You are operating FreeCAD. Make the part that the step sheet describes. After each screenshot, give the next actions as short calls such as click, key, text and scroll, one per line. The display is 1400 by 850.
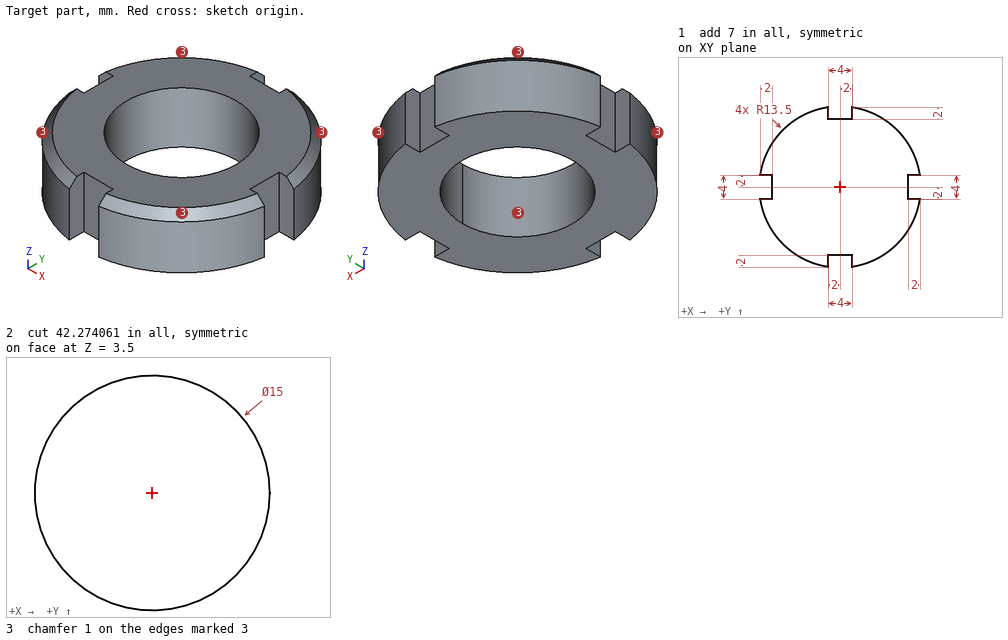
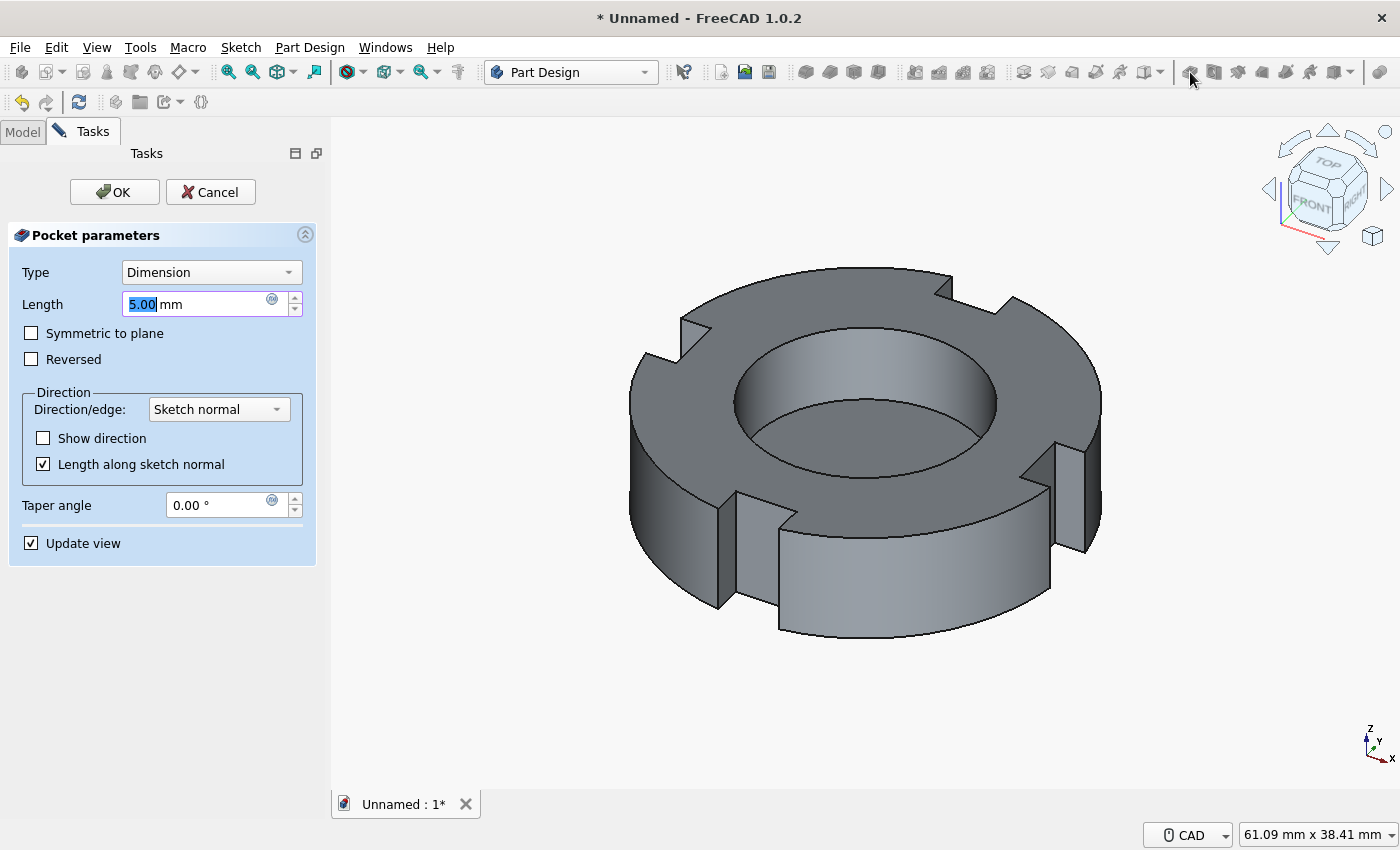
text(42.274061)
key(Tab)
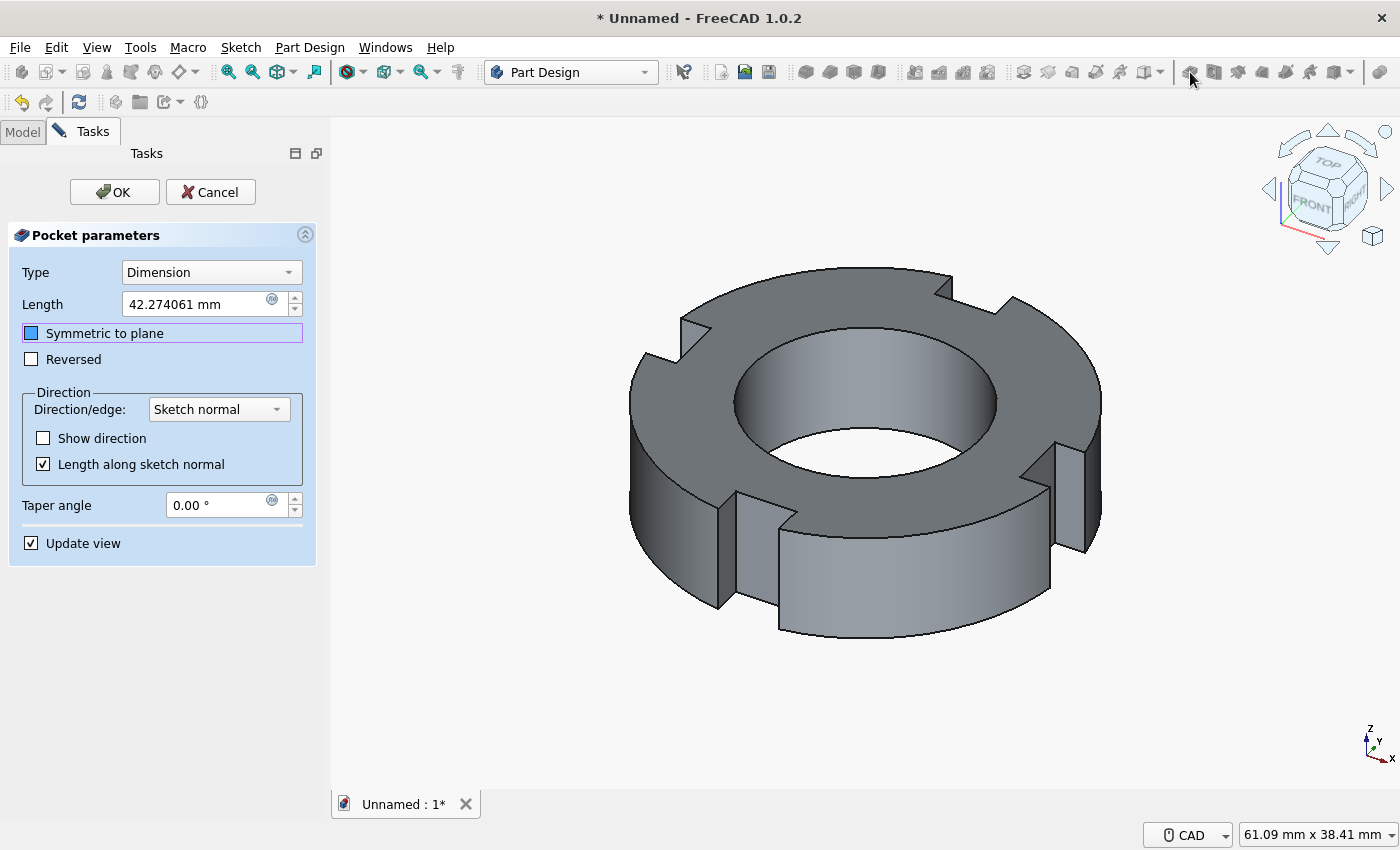
click(30, 333)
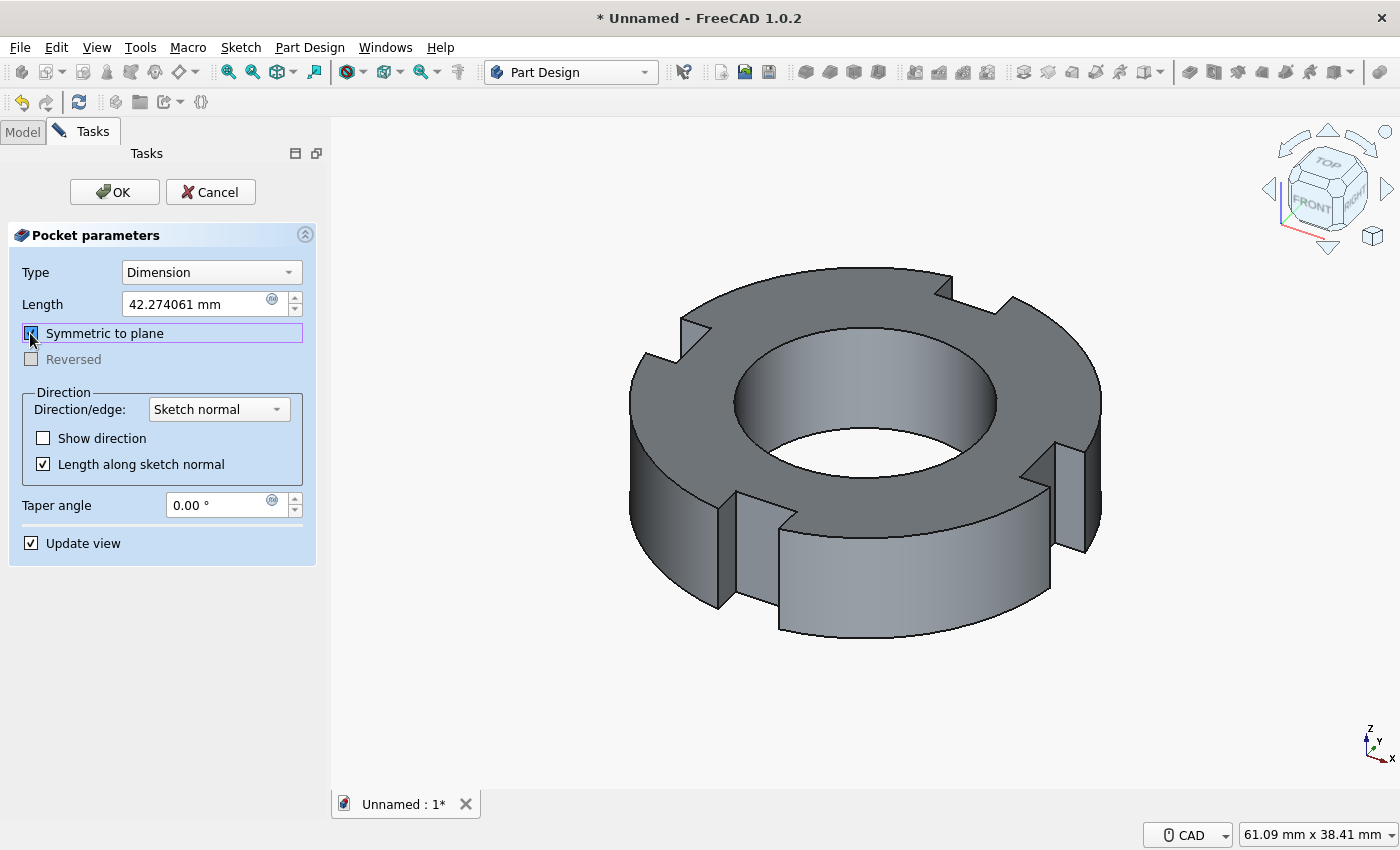
click(115, 192)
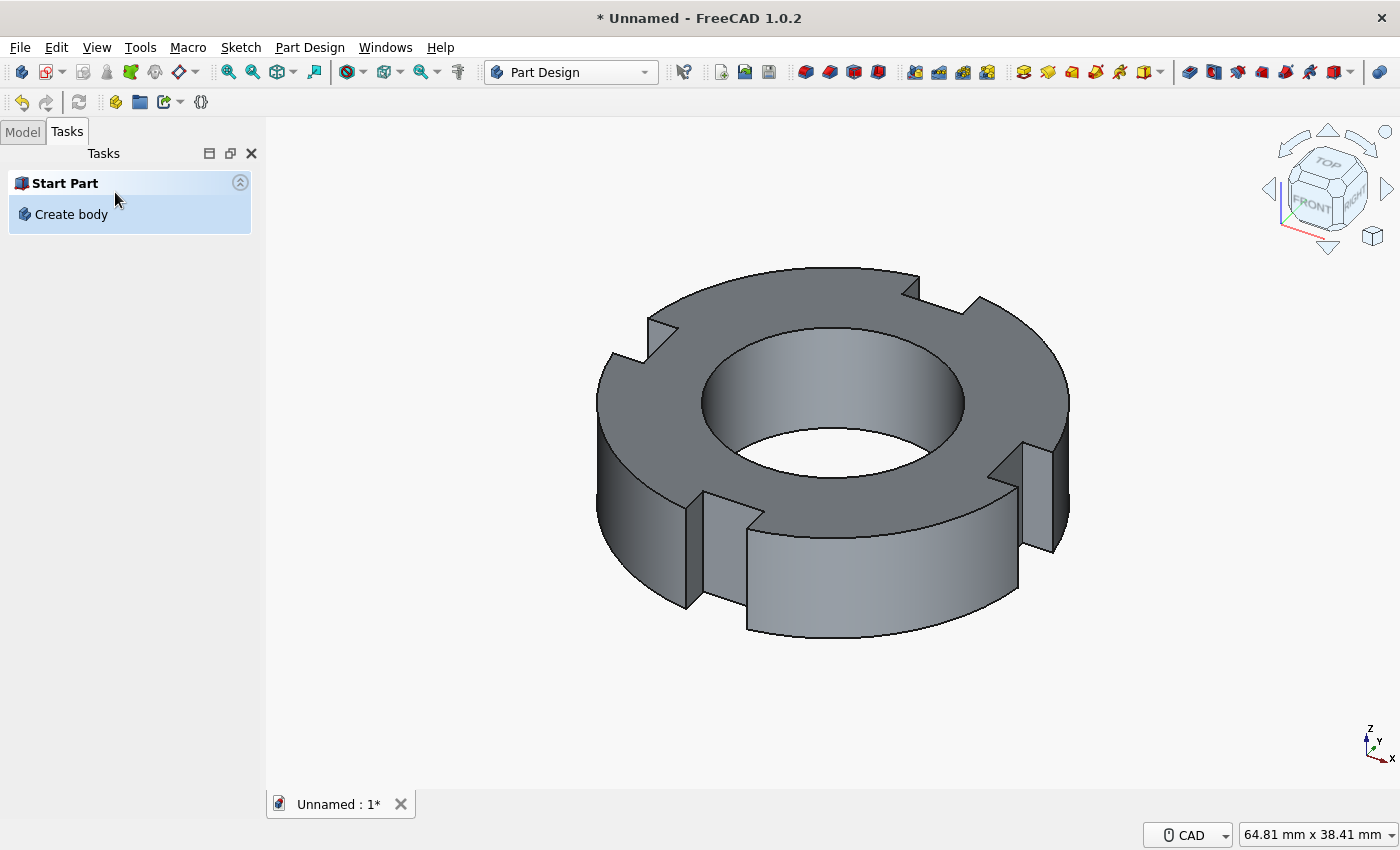
click(605, 437)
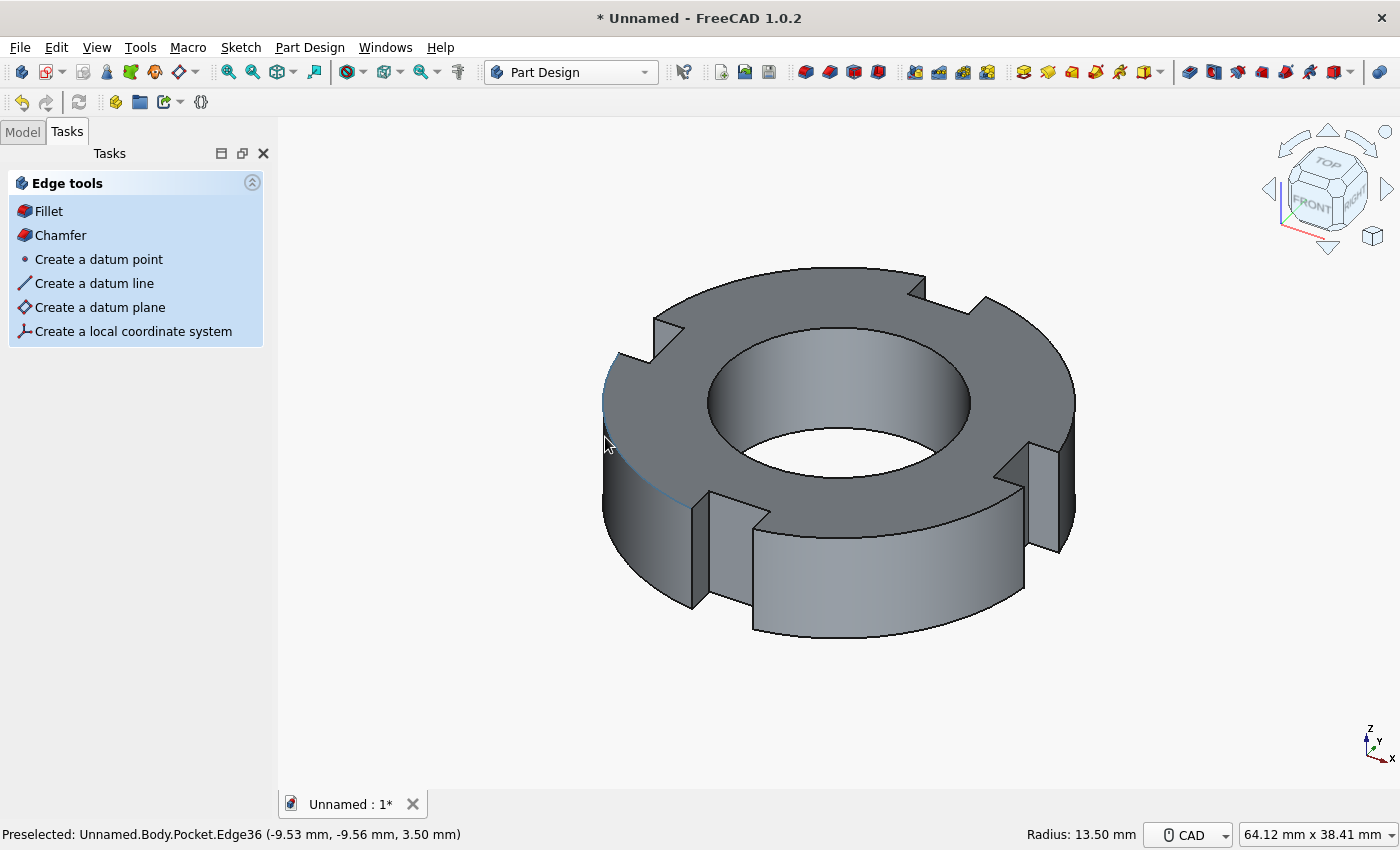
click(900, 533, ctrl)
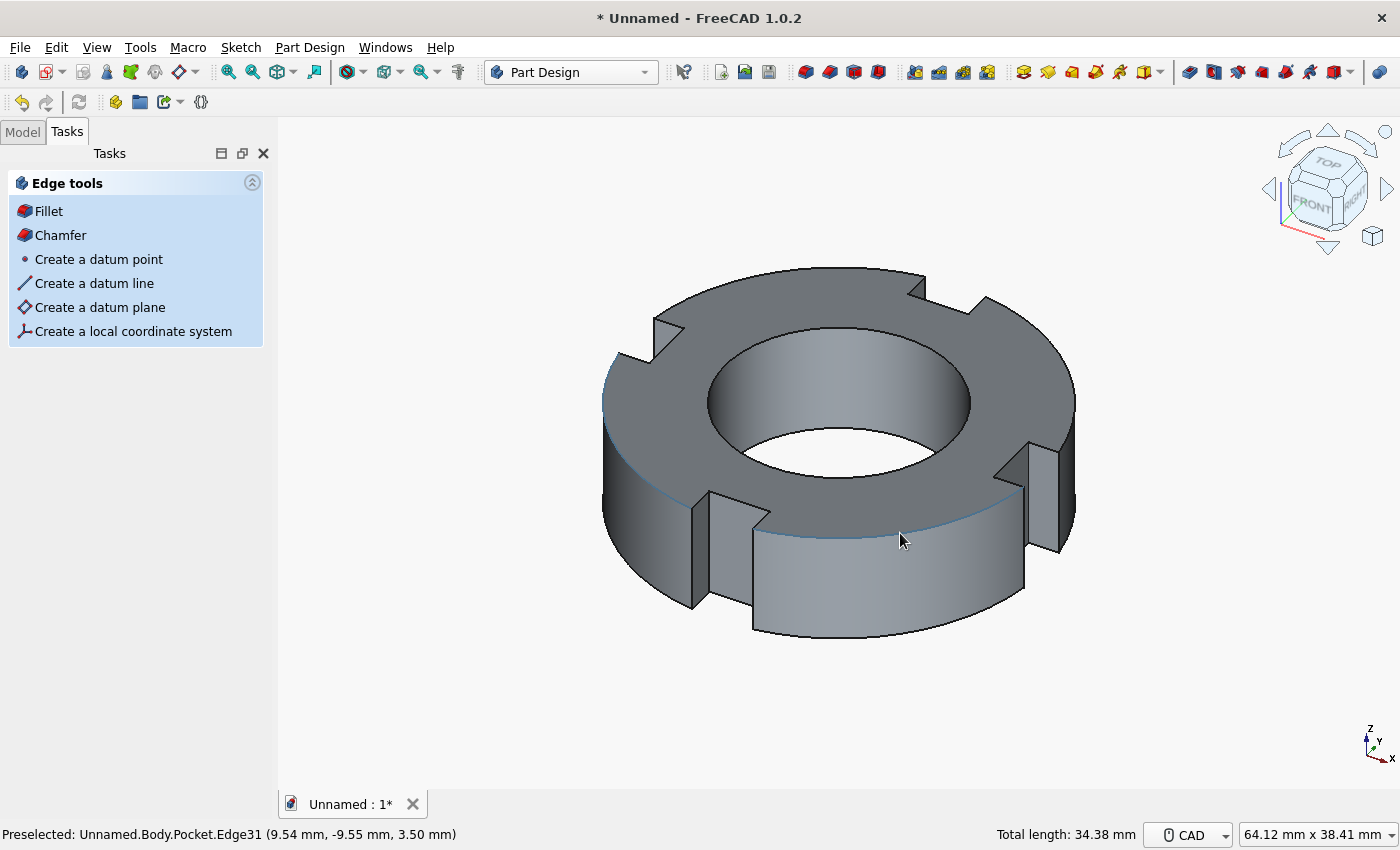
click(1058, 350, ctrl)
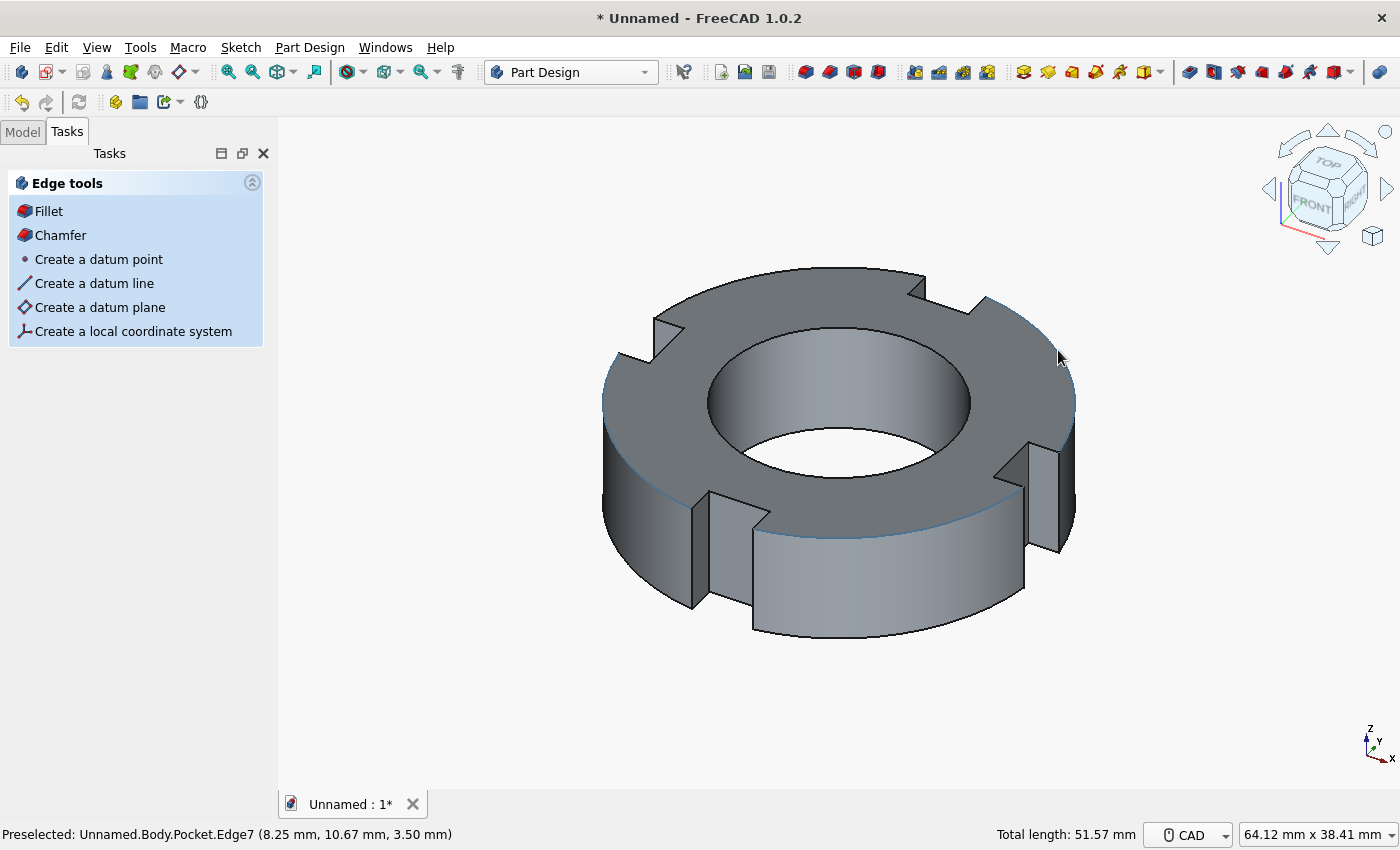
key(0)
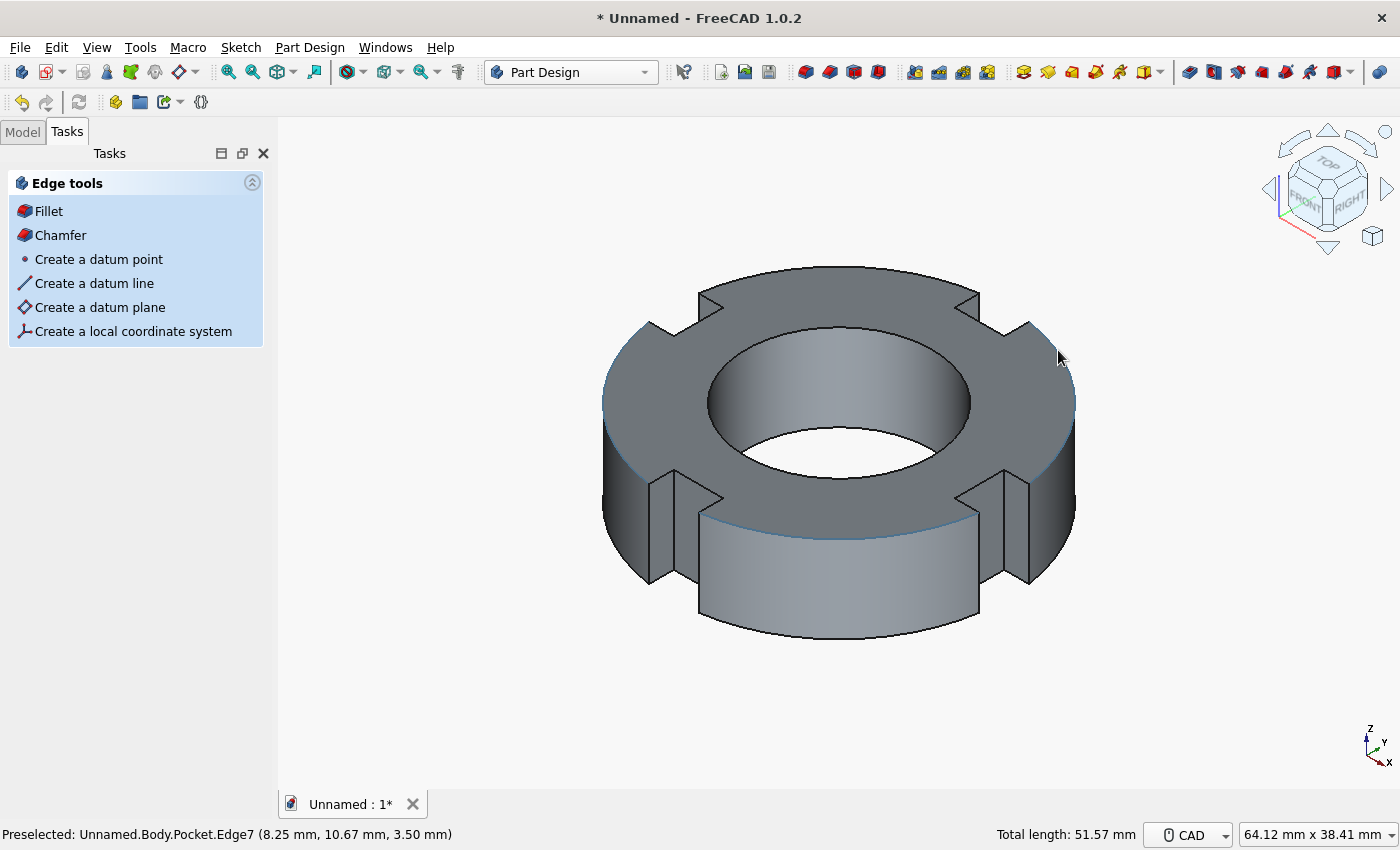
key(2)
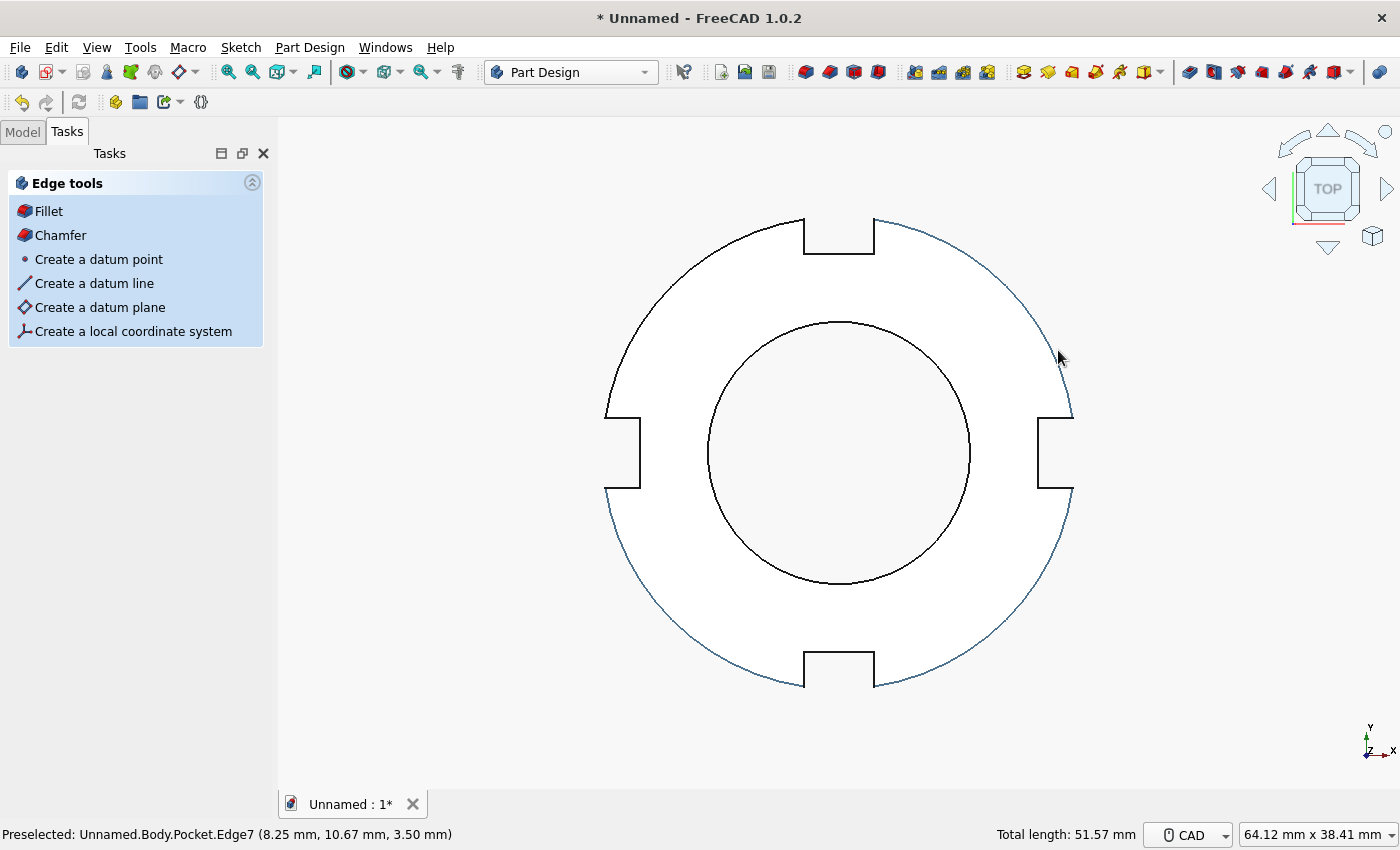
click(672, 285, ctrl)